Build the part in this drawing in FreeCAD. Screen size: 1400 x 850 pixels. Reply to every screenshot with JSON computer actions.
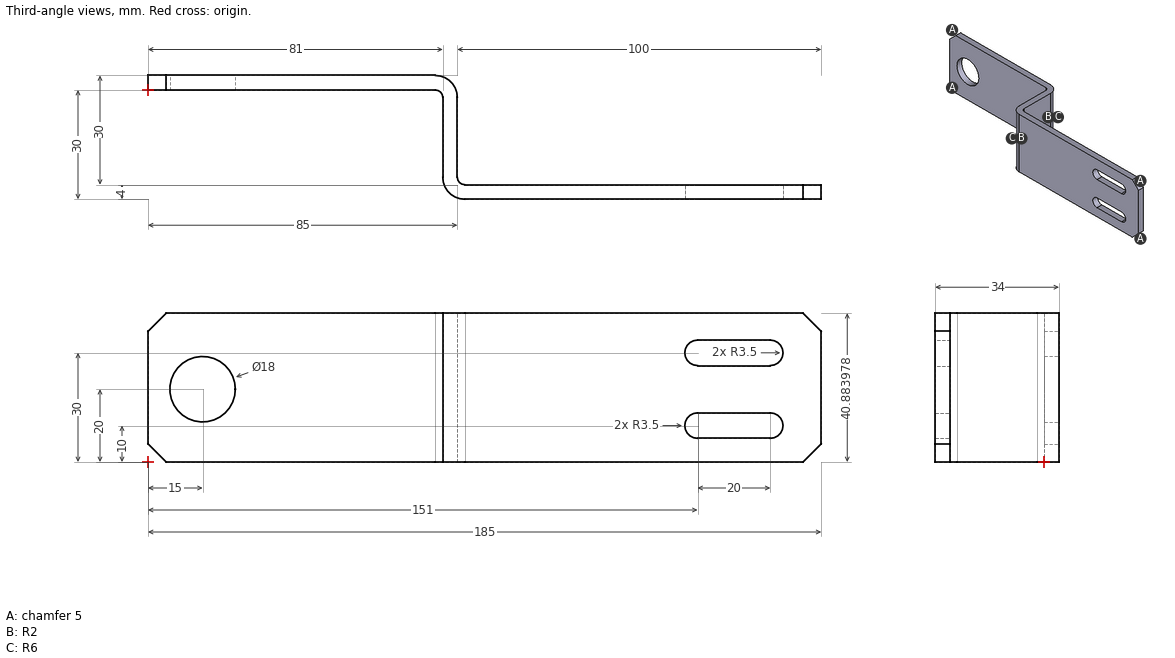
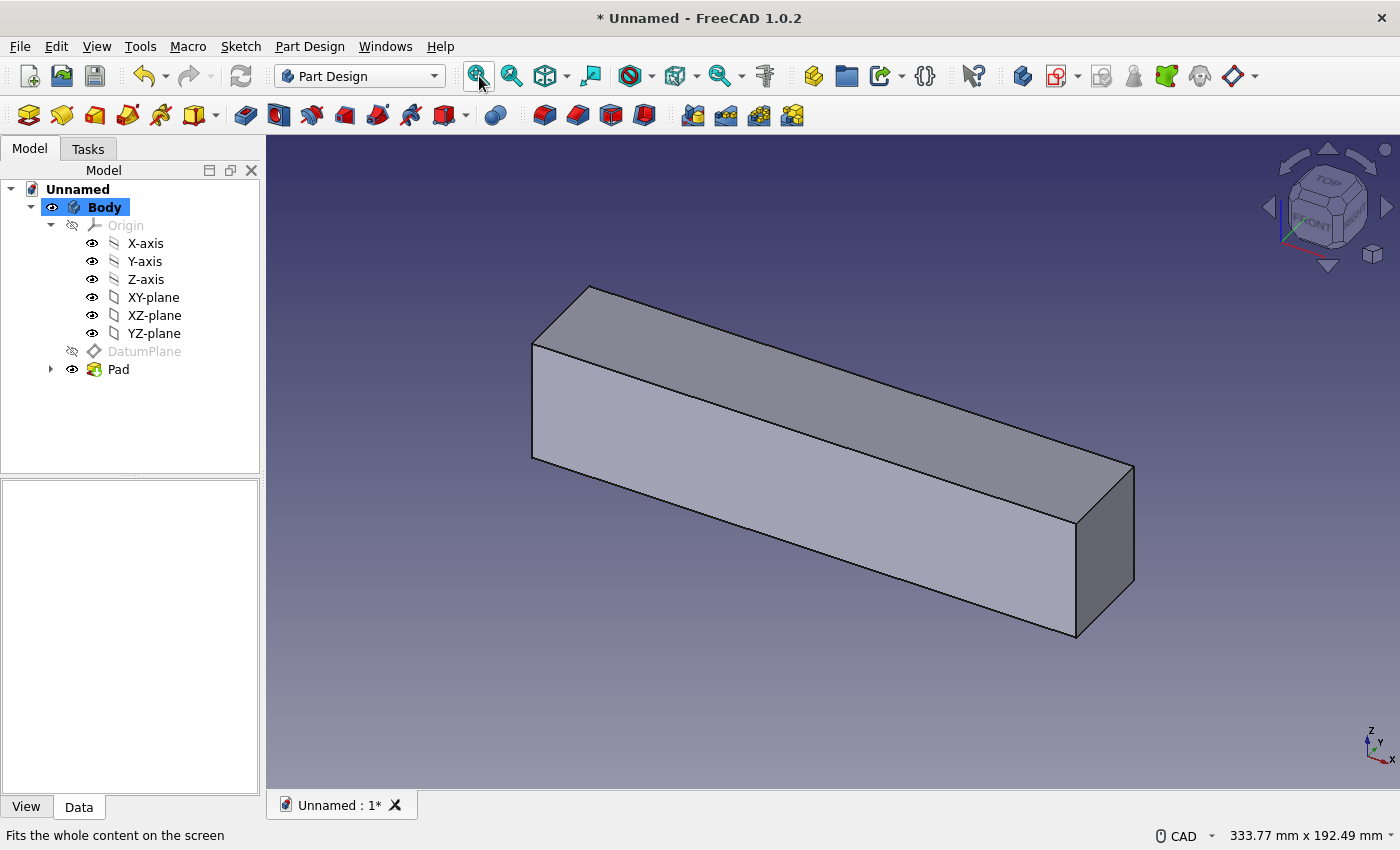
{"action": "key", "text": "5"}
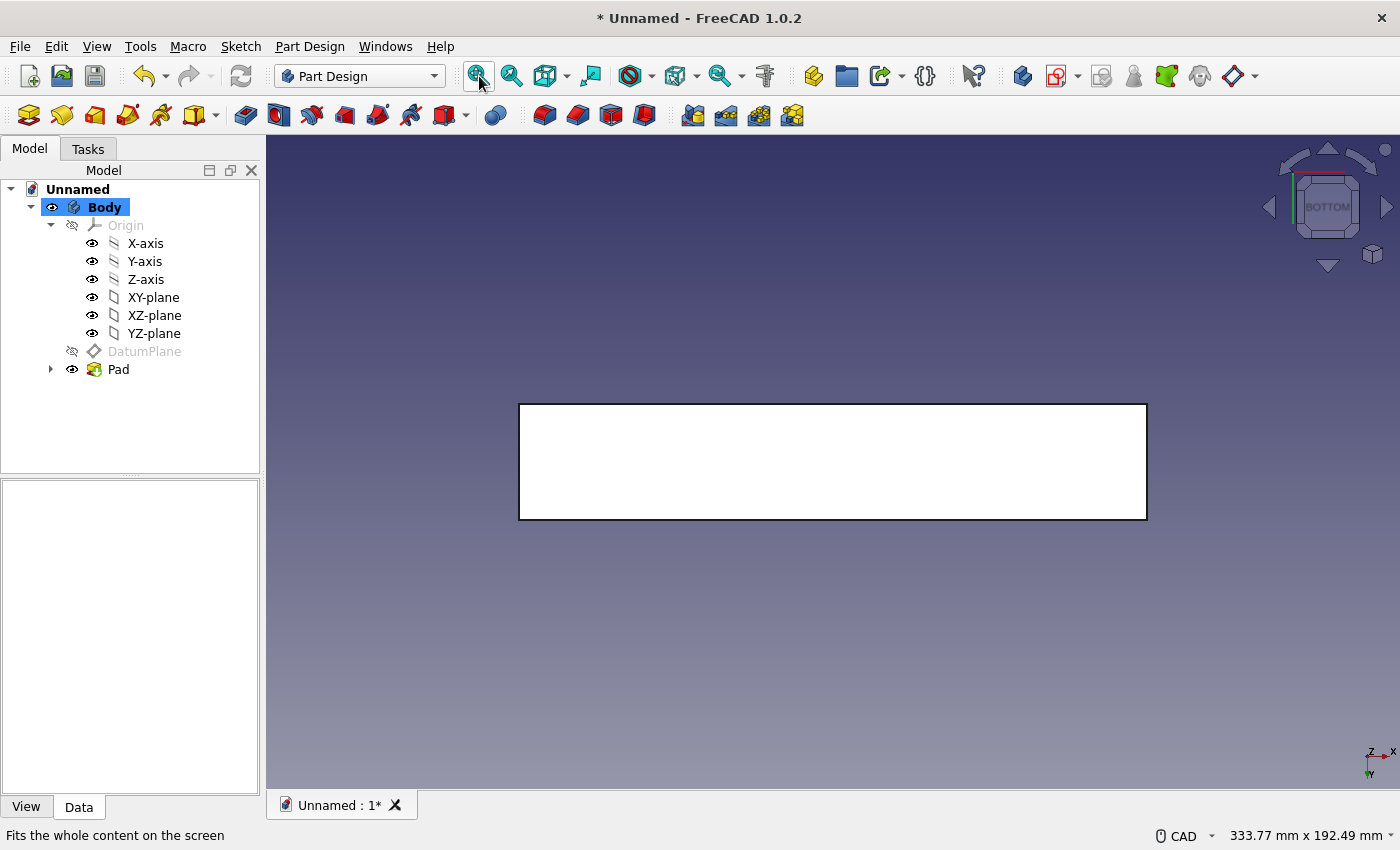
{"action": "left_click", "coordinate": [1013, 461]}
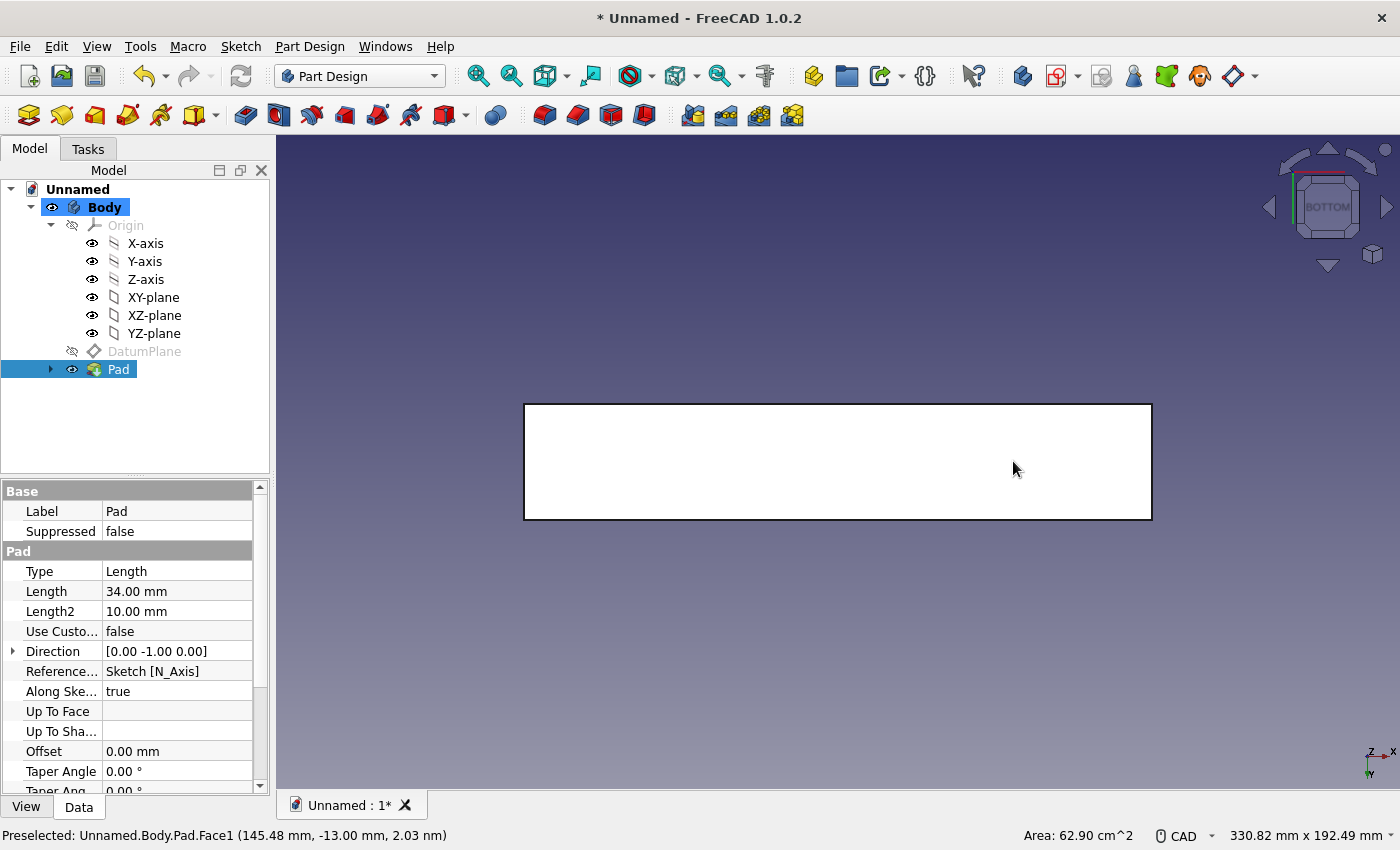
{"action": "left_click", "coordinate": [1056, 76]}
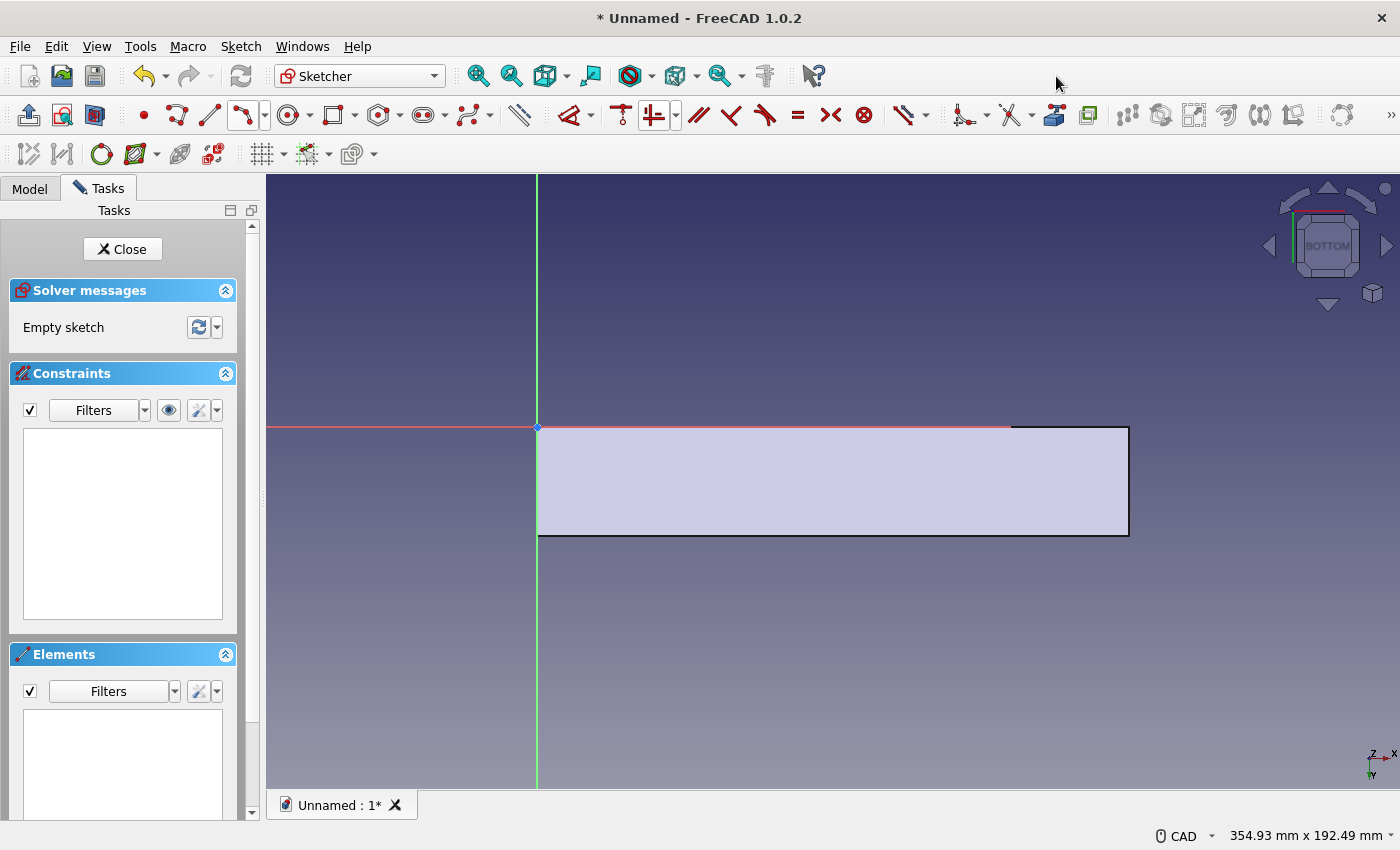
{"action": "left_click", "coordinate": [332, 116]}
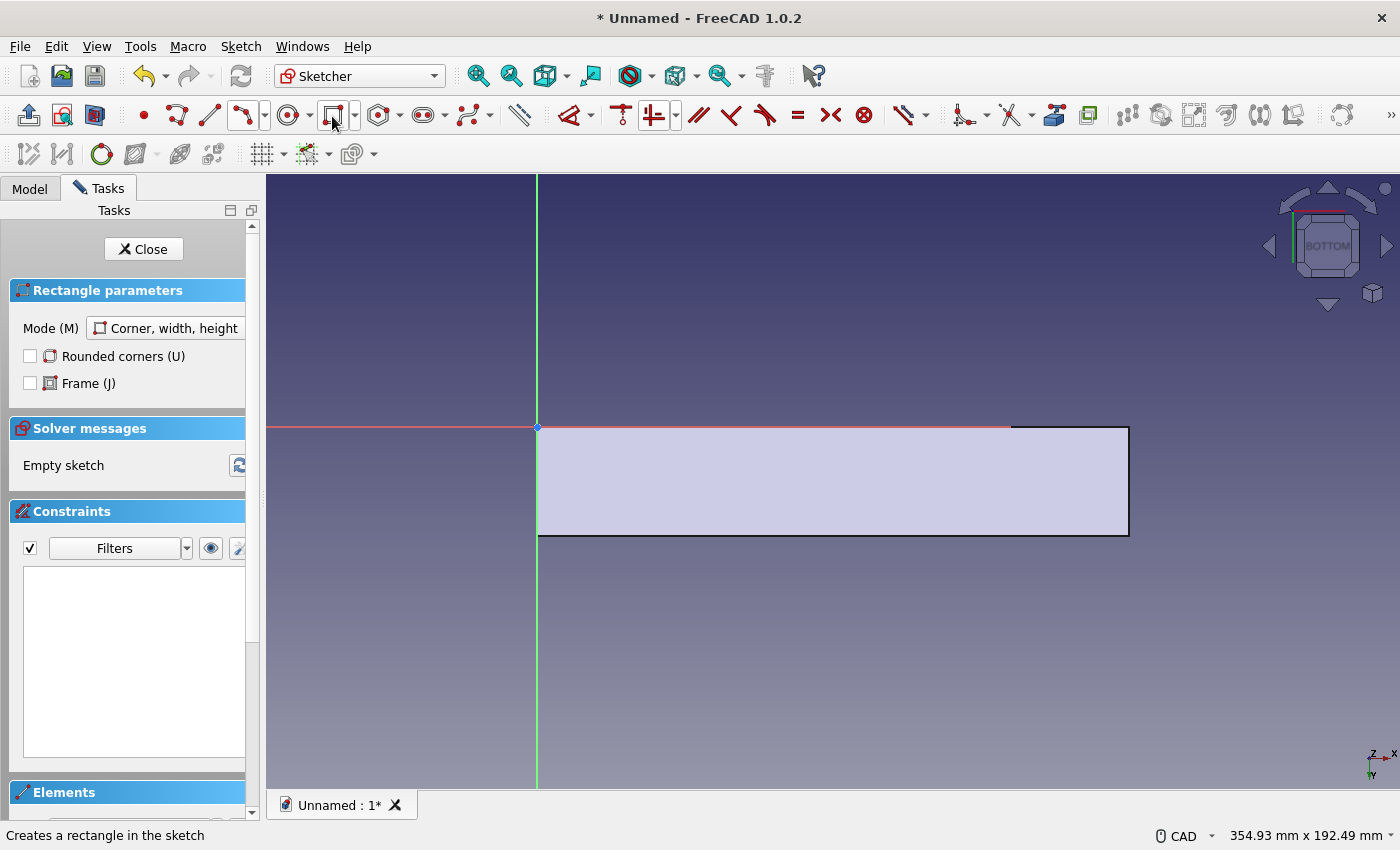
{"action": "scroll", "coordinate": [809, 440], "scroll_direction": "up", "scroll_amount": 2}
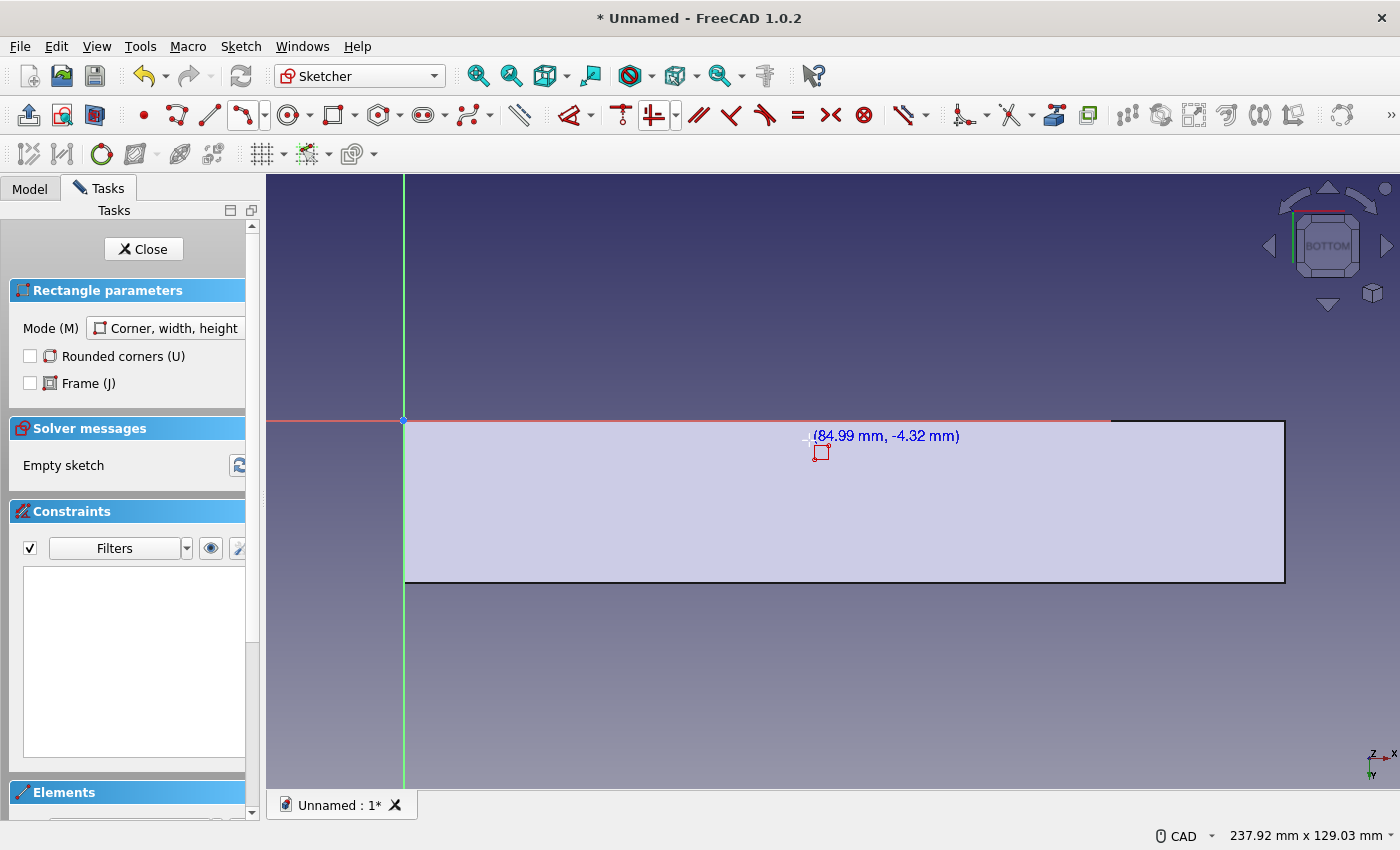
{"action": "left_click", "coordinate": [809, 440]}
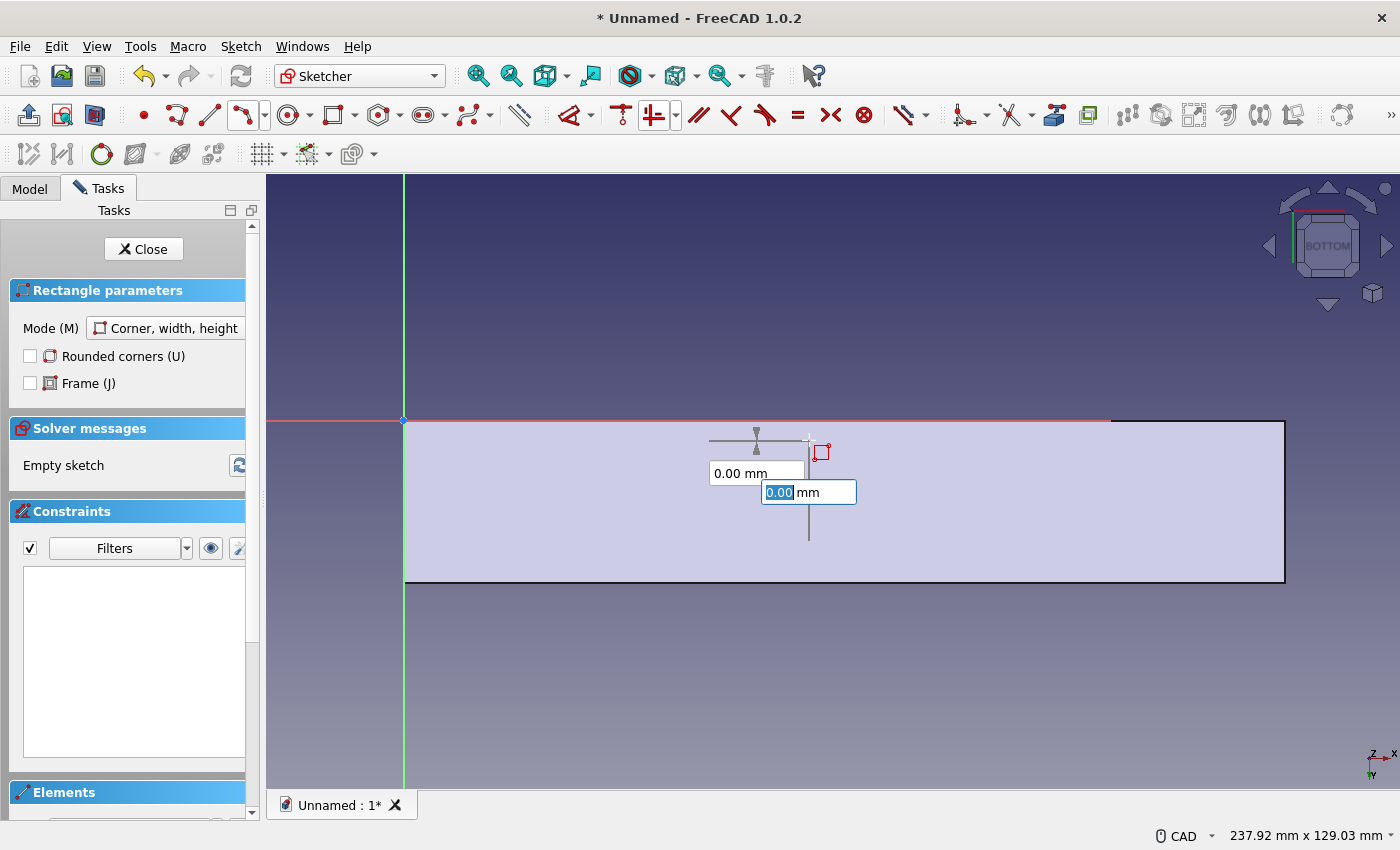
{"action": "scroll", "coordinate": [403, 390], "scroll_direction": "down", "scroll_amount": 1}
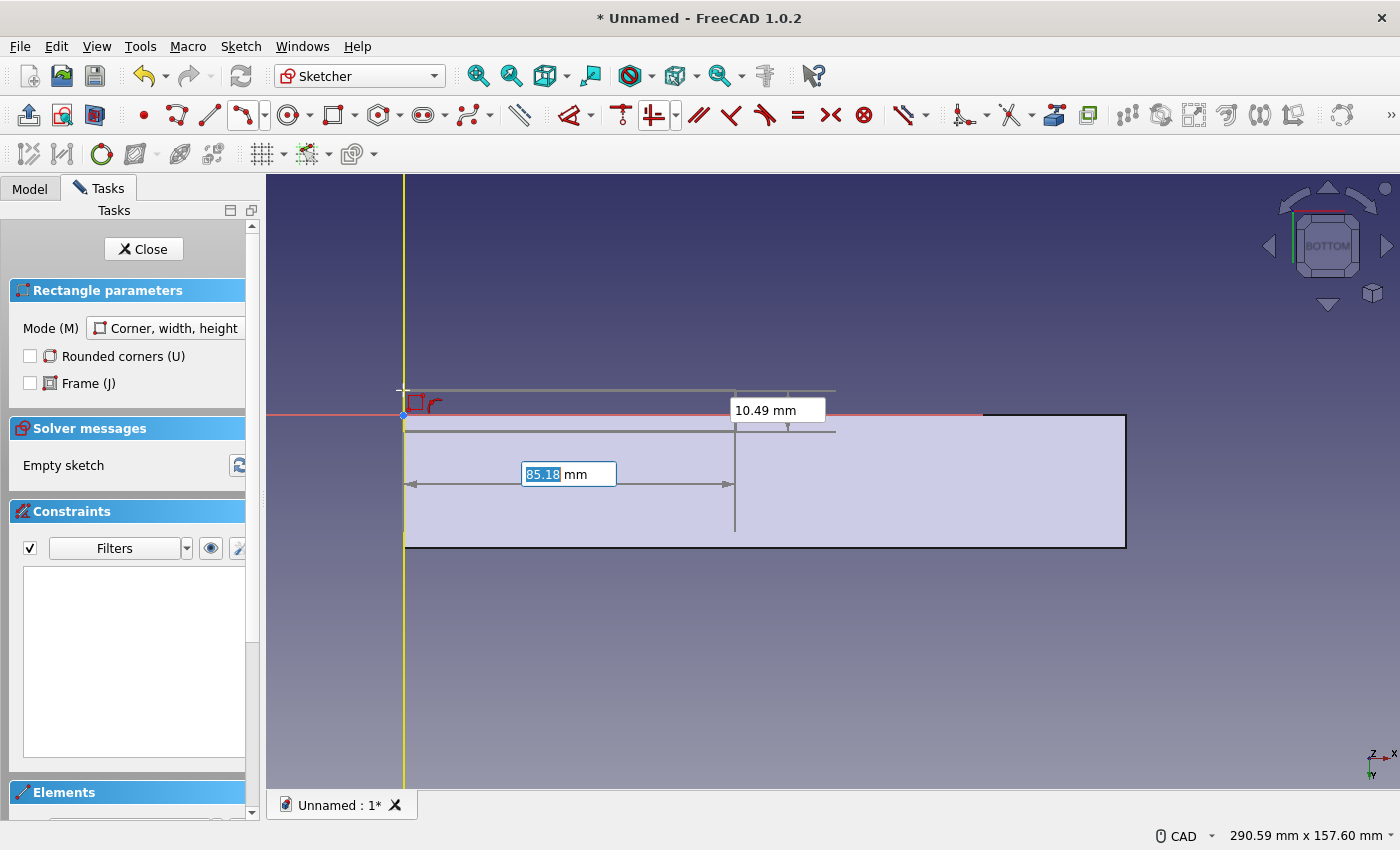
{"action": "left_click", "coordinate": [1126, 548]}
{"action": "key", "text": "Escape"}